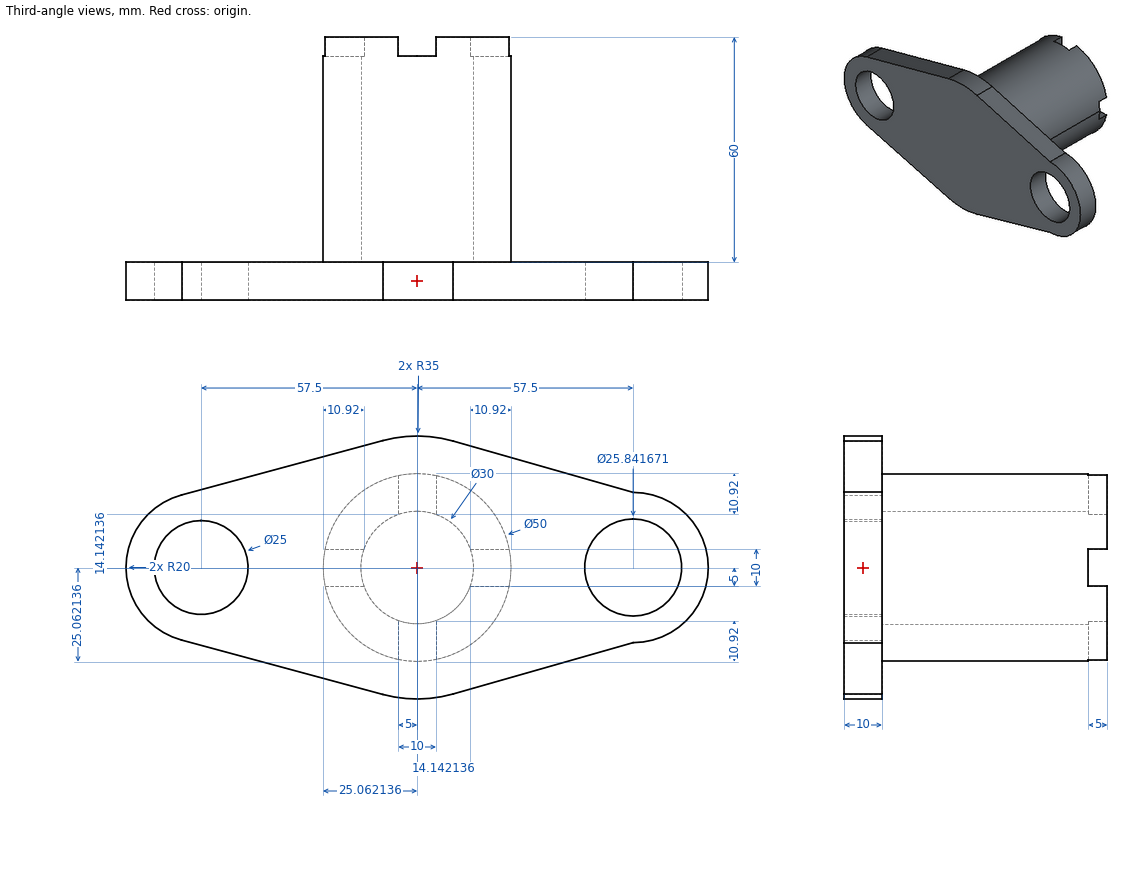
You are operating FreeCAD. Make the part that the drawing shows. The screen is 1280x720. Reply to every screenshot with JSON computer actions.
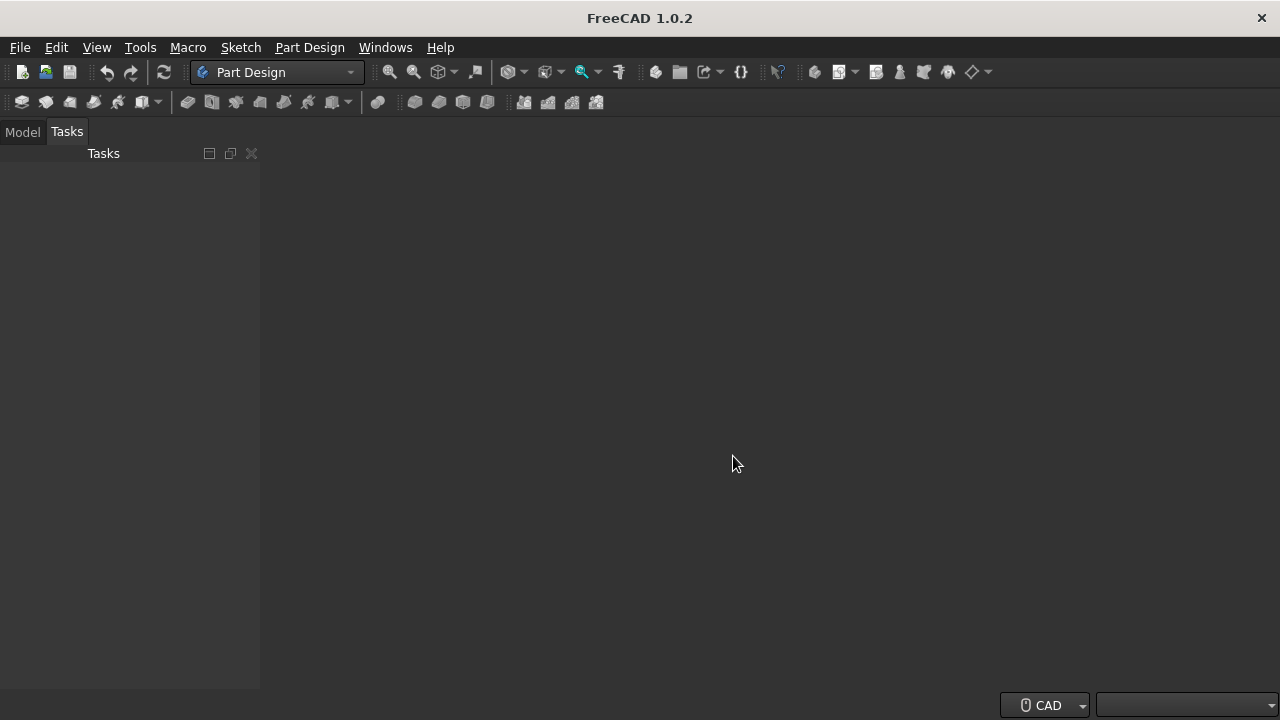
{"action": "key", "text": "ctrl+n"}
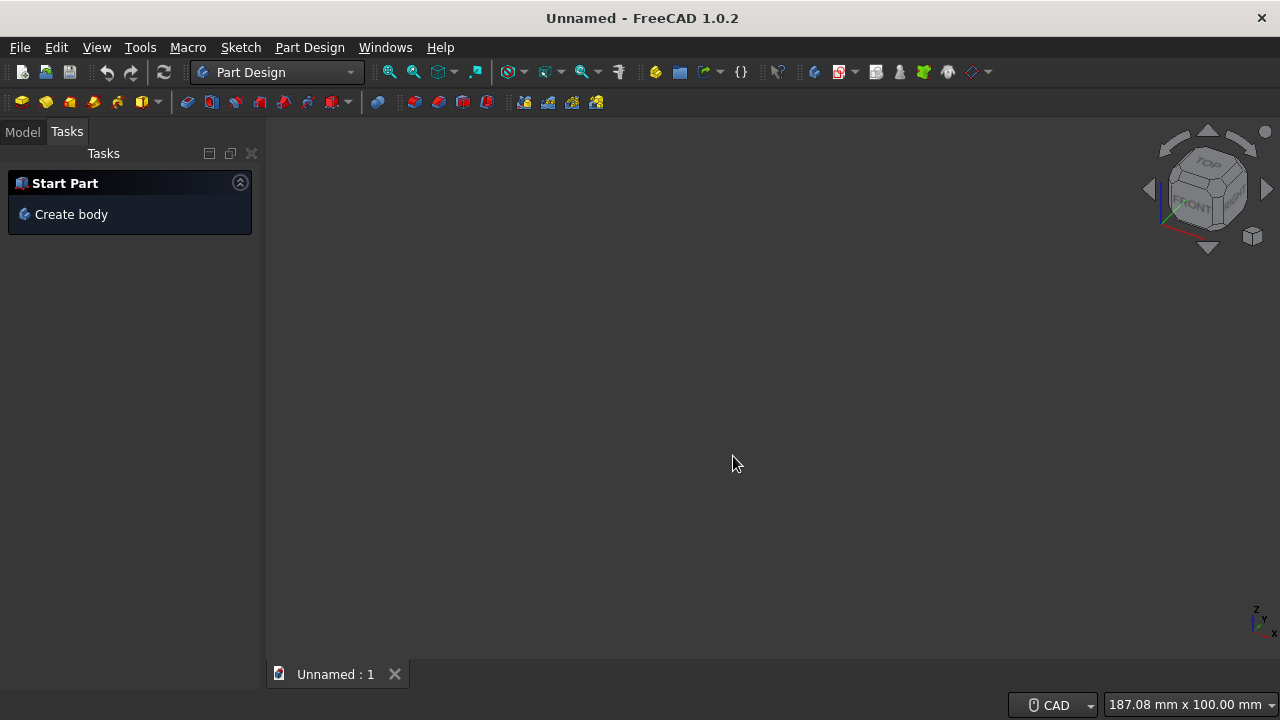
{"action": "left_click", "coordinate": [840, 72]}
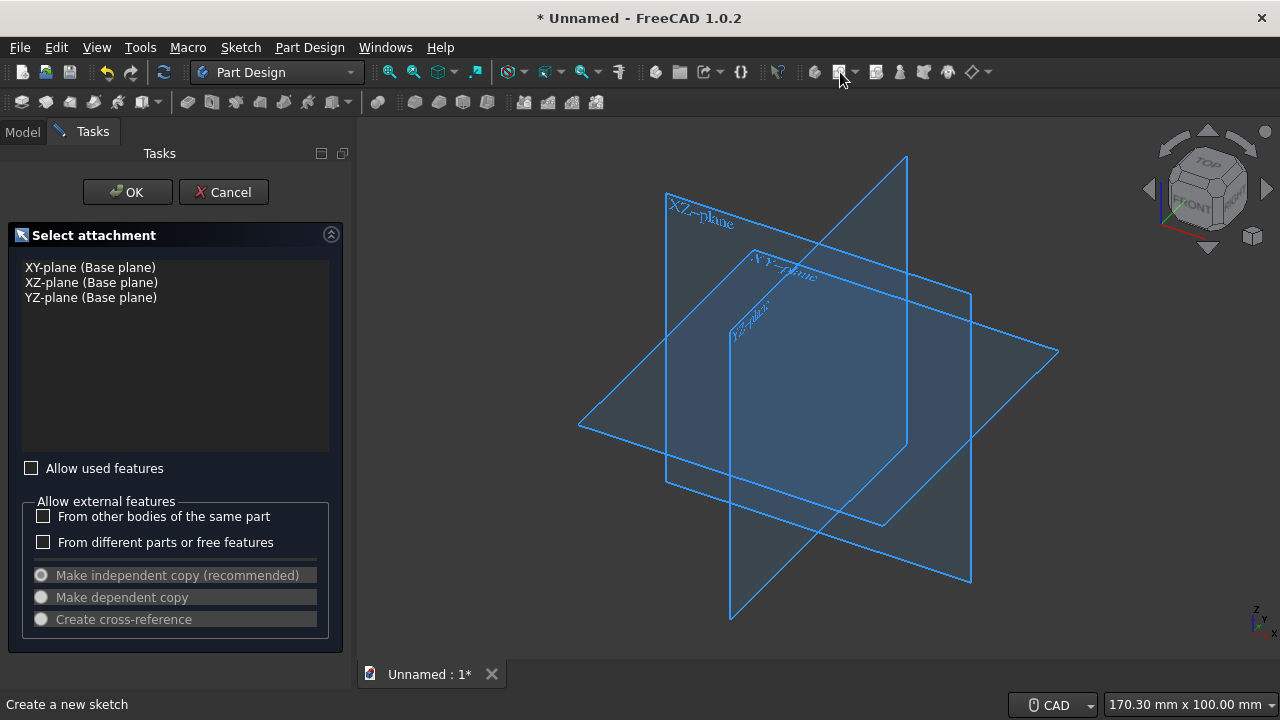
{"action": "left_click", "coordinate": [82, 282]}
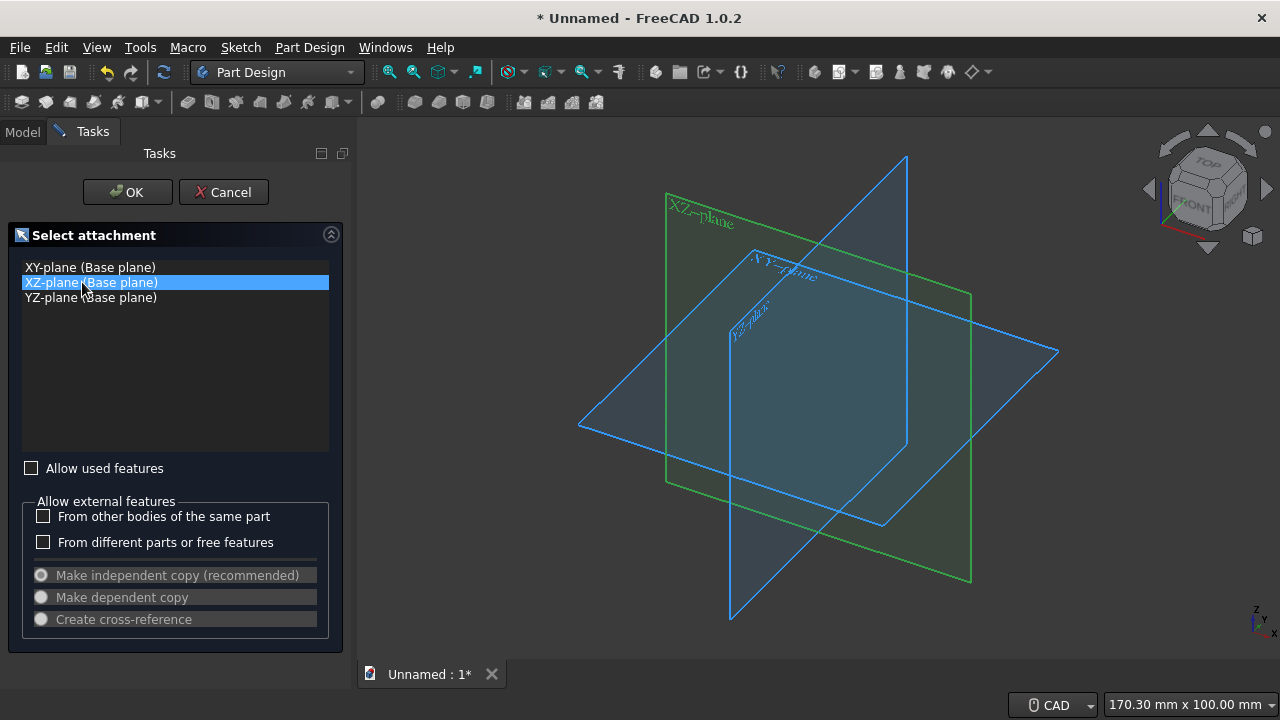
{"action": "left_click", "coordinate": [128, 192]}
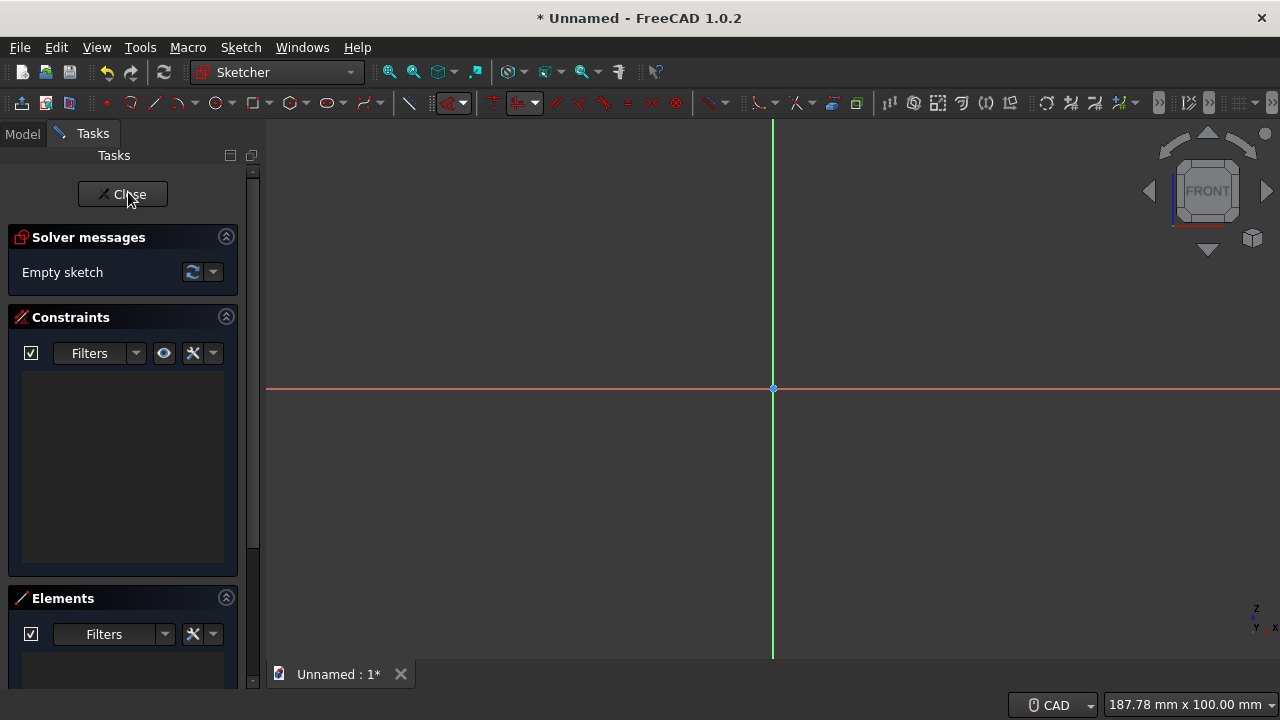
{"action": "scroll", "coordinate": [565, 389], "scroll_direction": "down", "scroll_amount": 2}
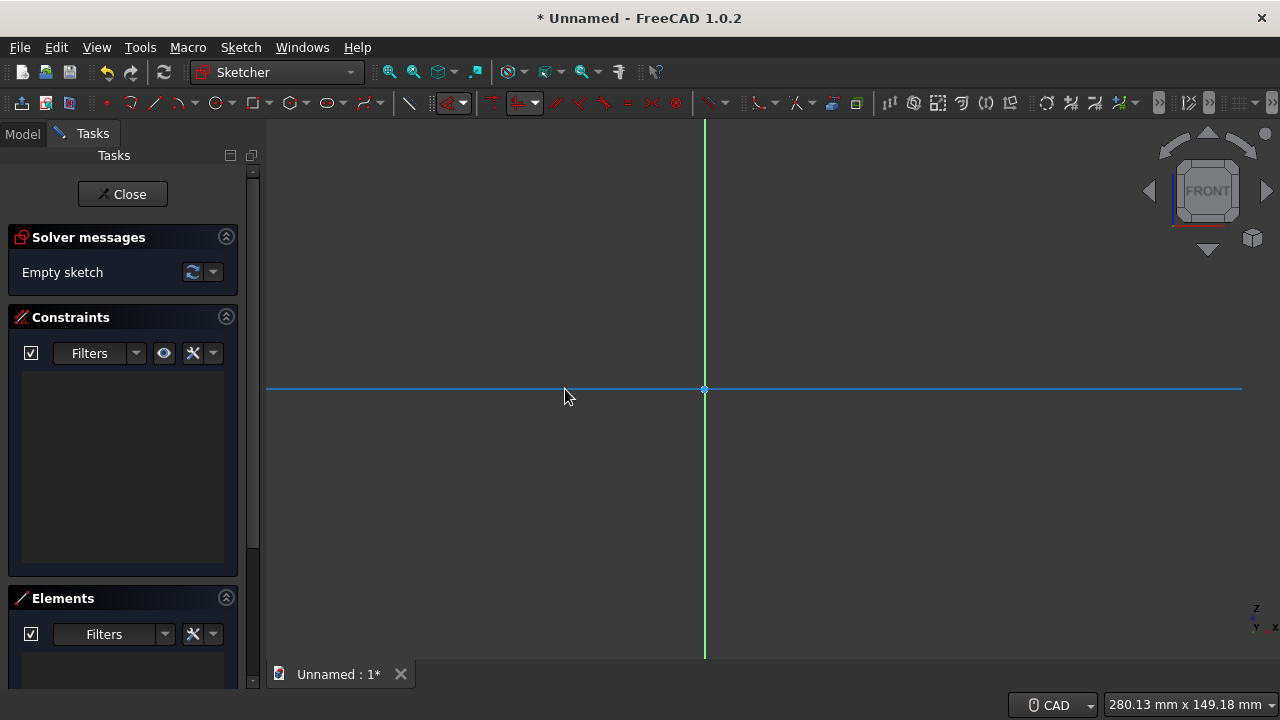
{"action": "key", "text": "g l"}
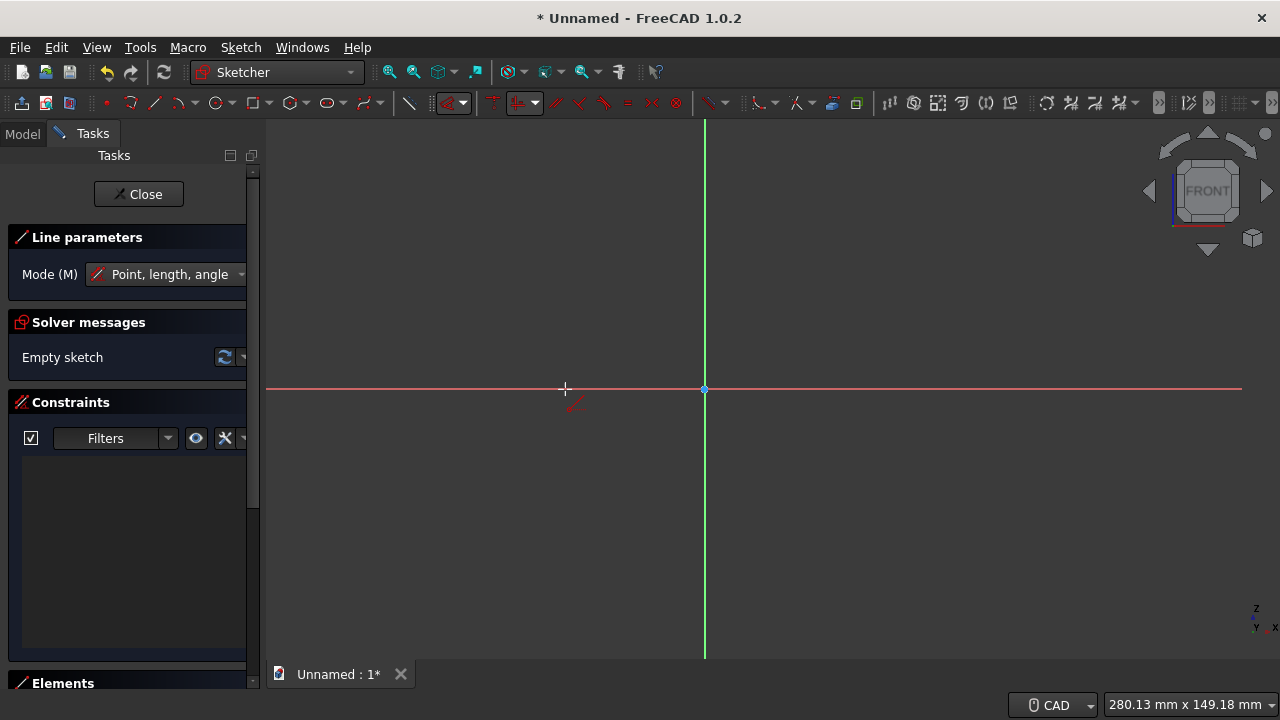
{"action": "left_click", "coordinate": [671, 511]}
{"action": "left_click", "coordinate": [478, 459]}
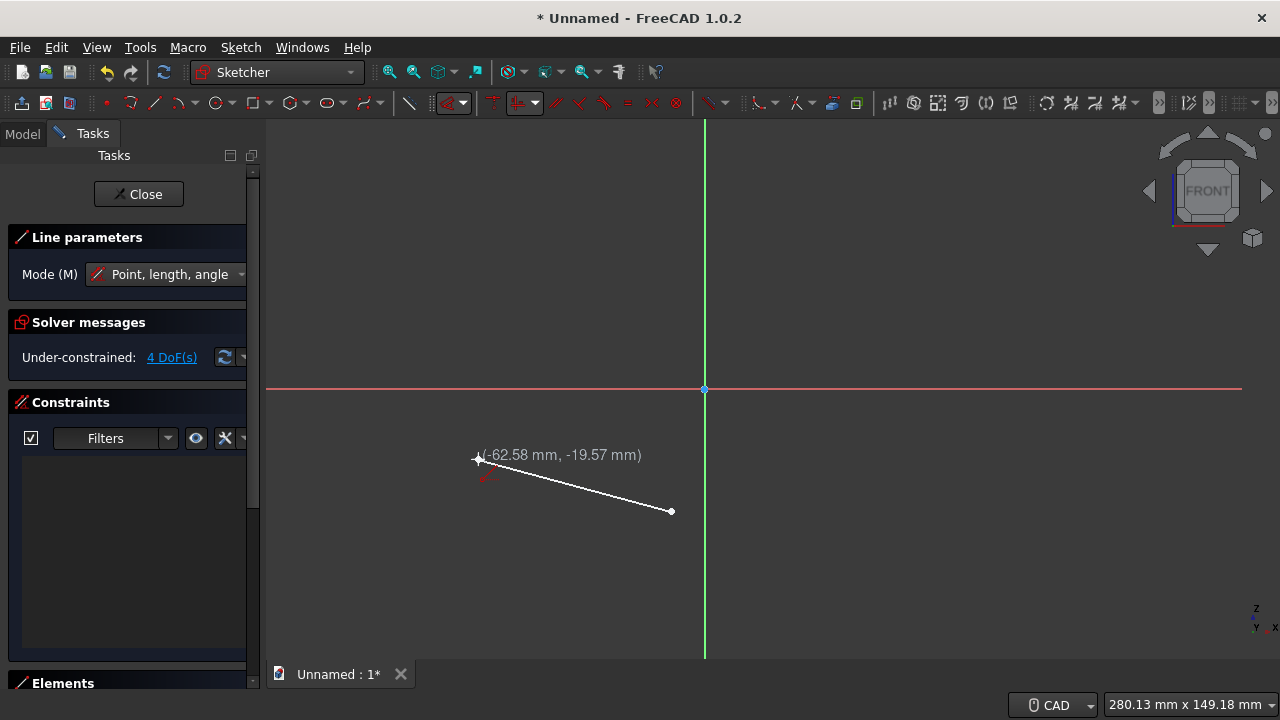
{"action": "left_click", "coordinate": [478, 319]}
{"action": "left_click", "coordinate": [671, 267]}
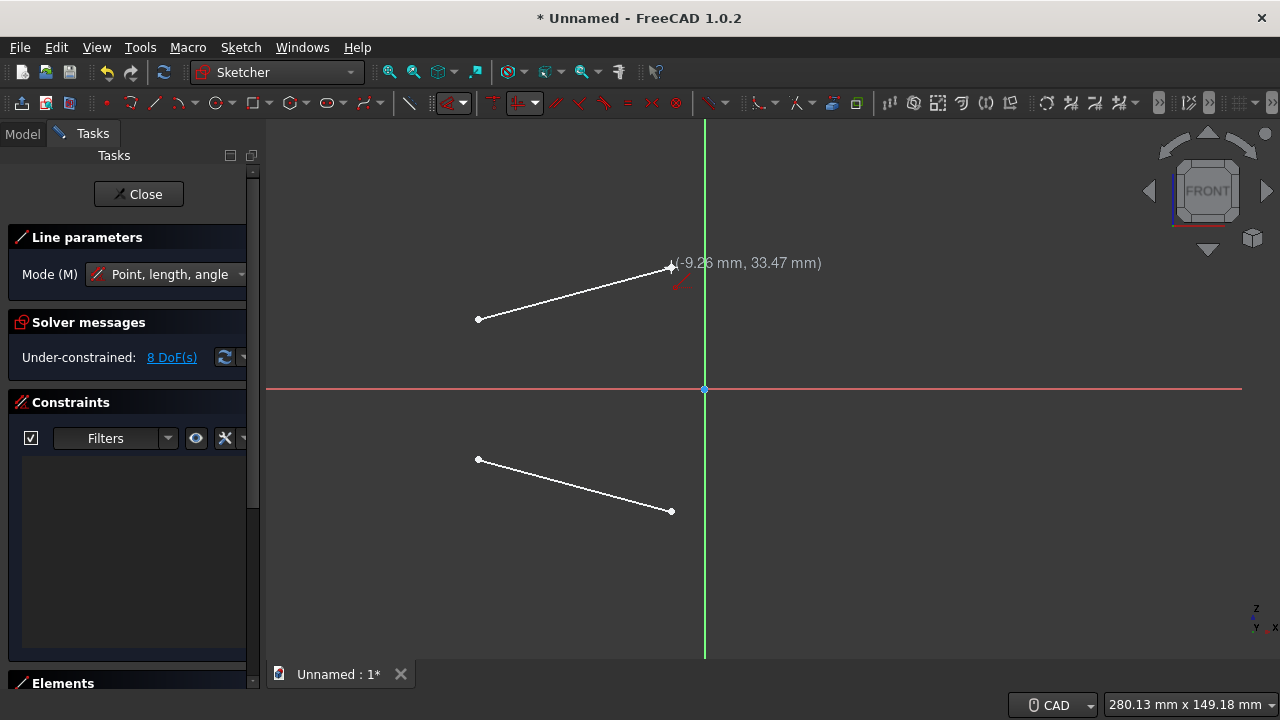
{"action": "left_click", "coordinate": [739, 267]}
{"action": "left_click", "coordinate": [913, 317]}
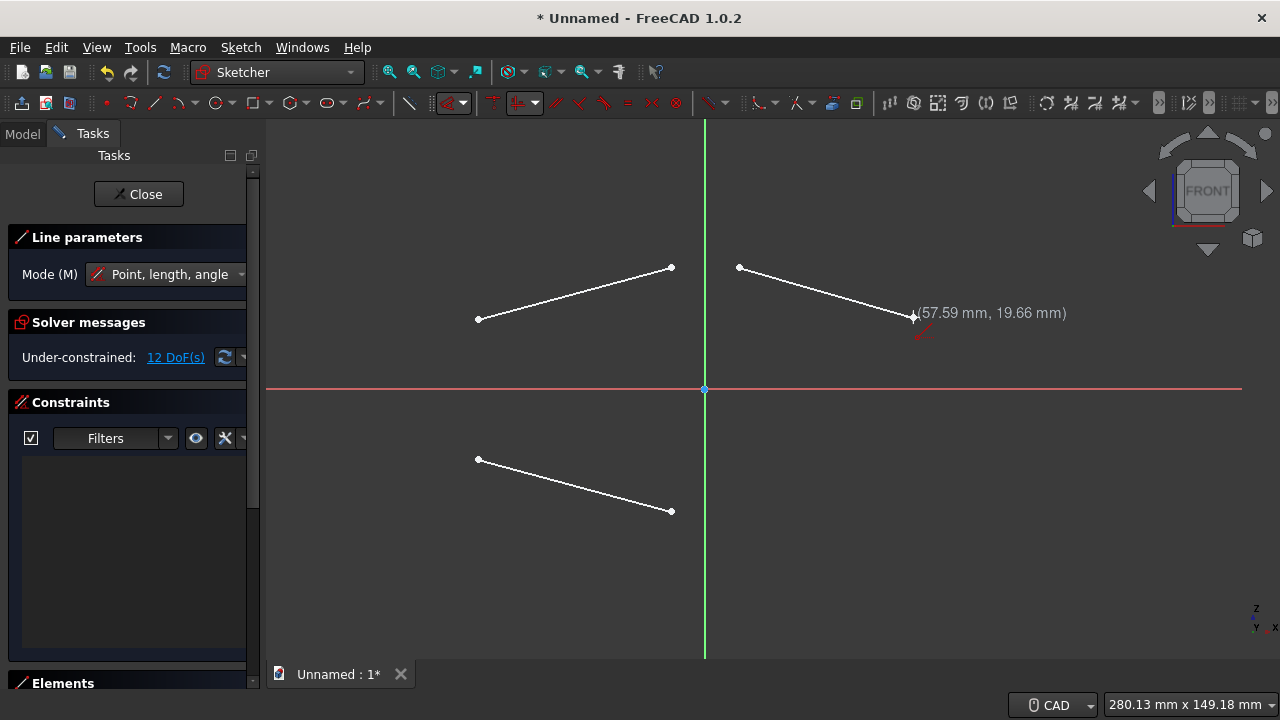
{"action": "left_click", "coordinate": [913, 462]}
{"action": "left_click", "coordinate": [739, 511]}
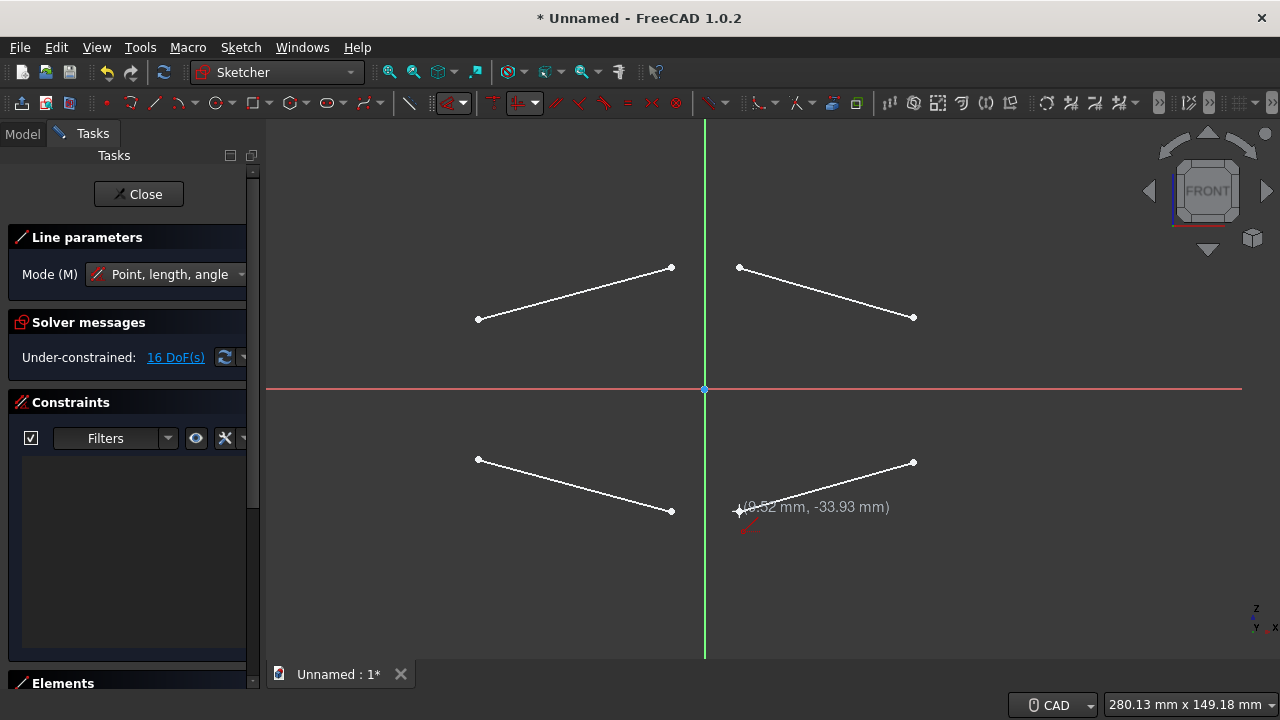
{"action": "key", "text": "g 3 a"}